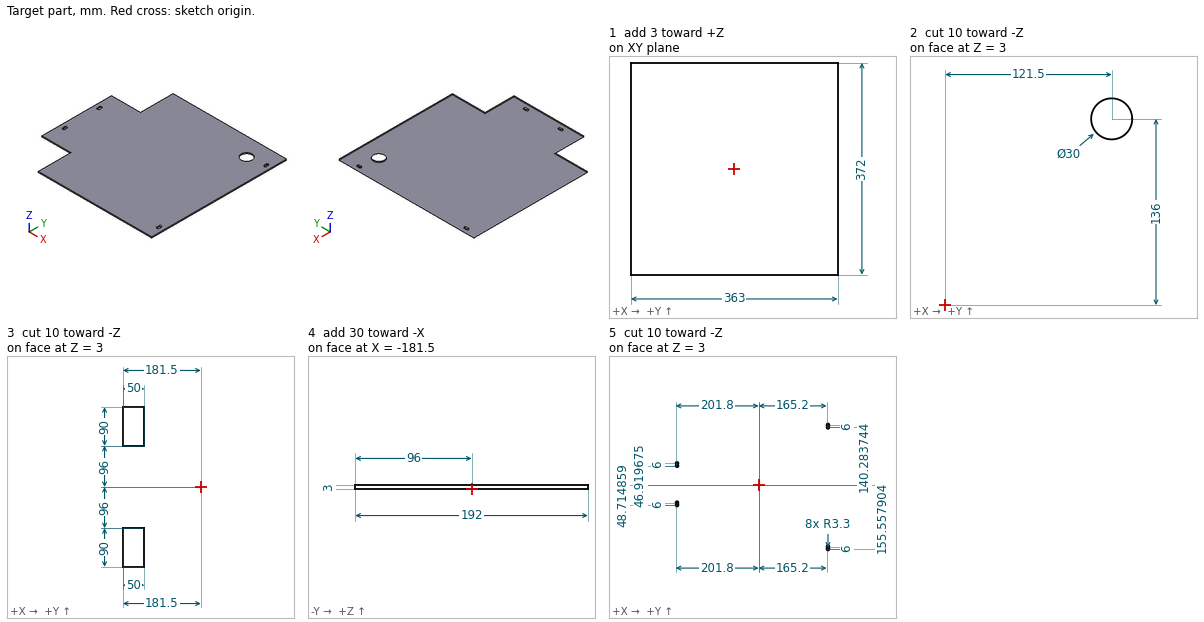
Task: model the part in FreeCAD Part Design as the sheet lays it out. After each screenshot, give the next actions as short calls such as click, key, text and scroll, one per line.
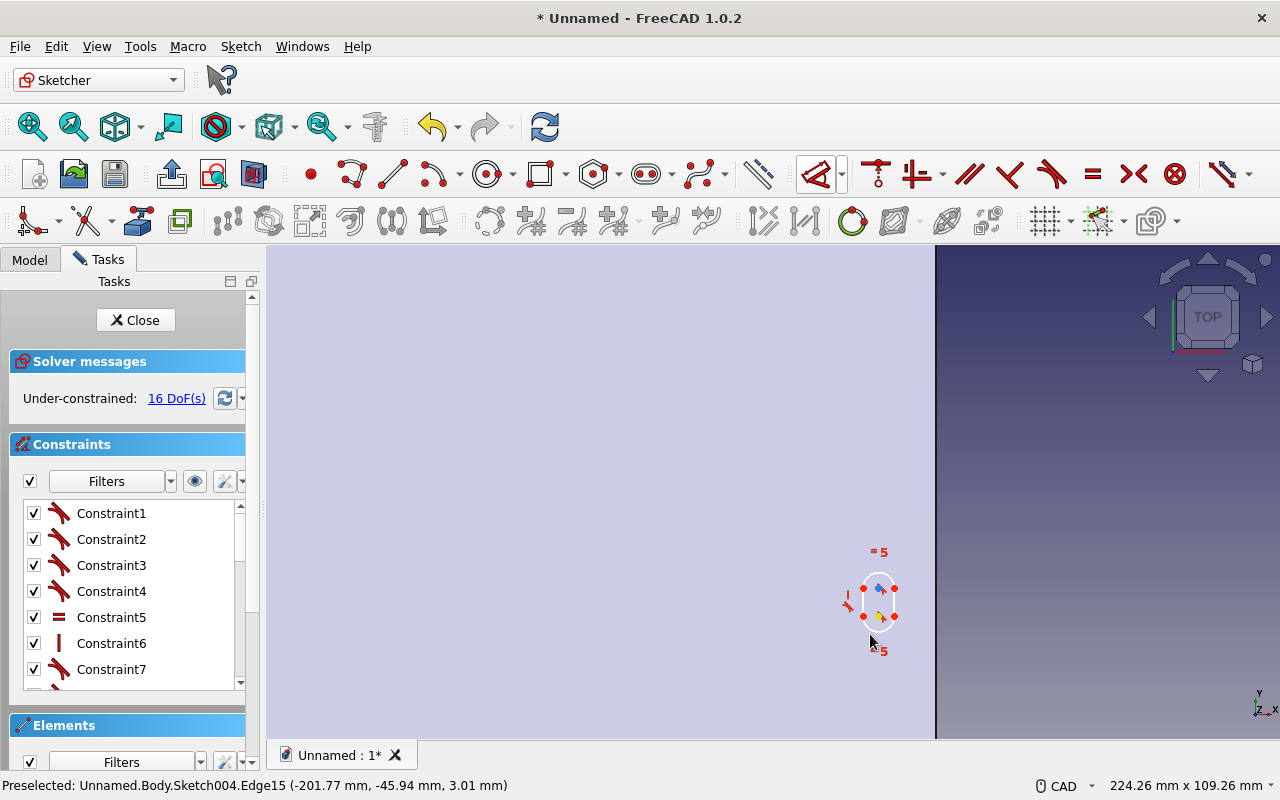
click(870, 629)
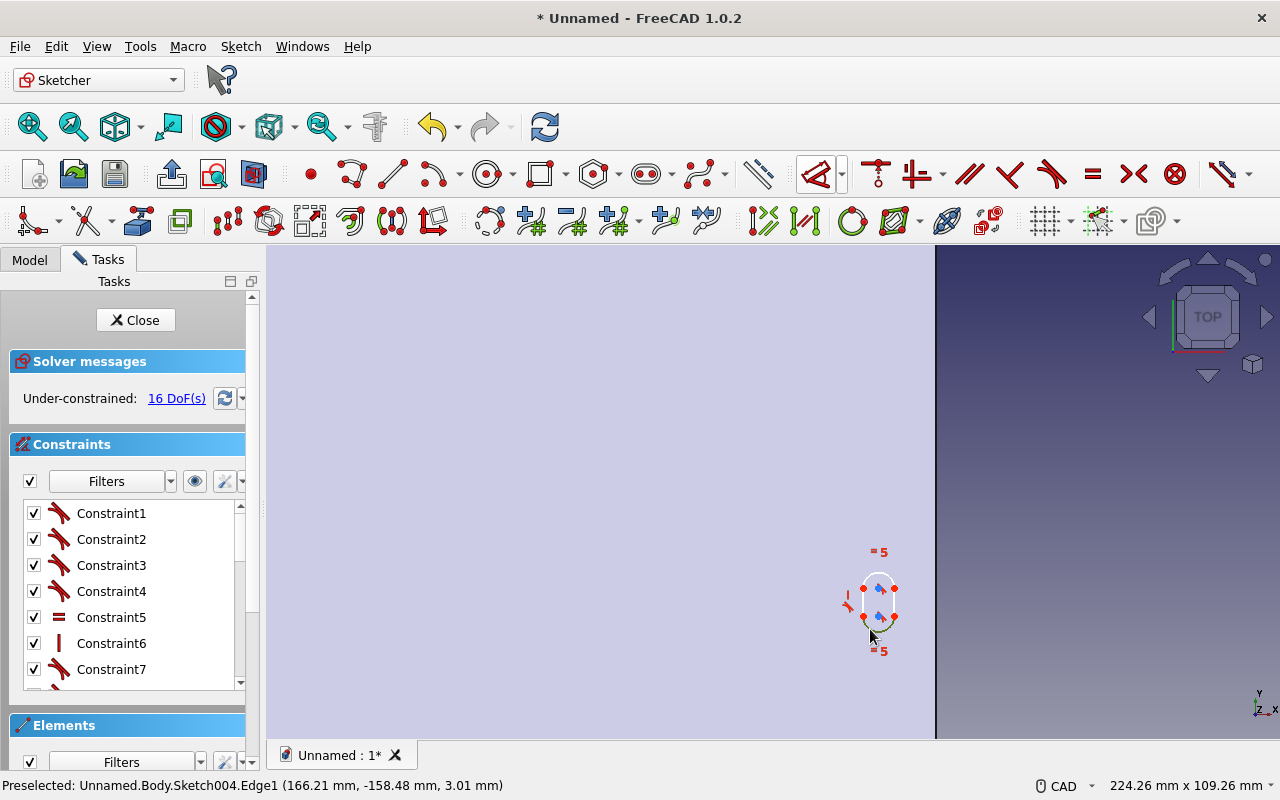
scroll(871, 634, down, 8)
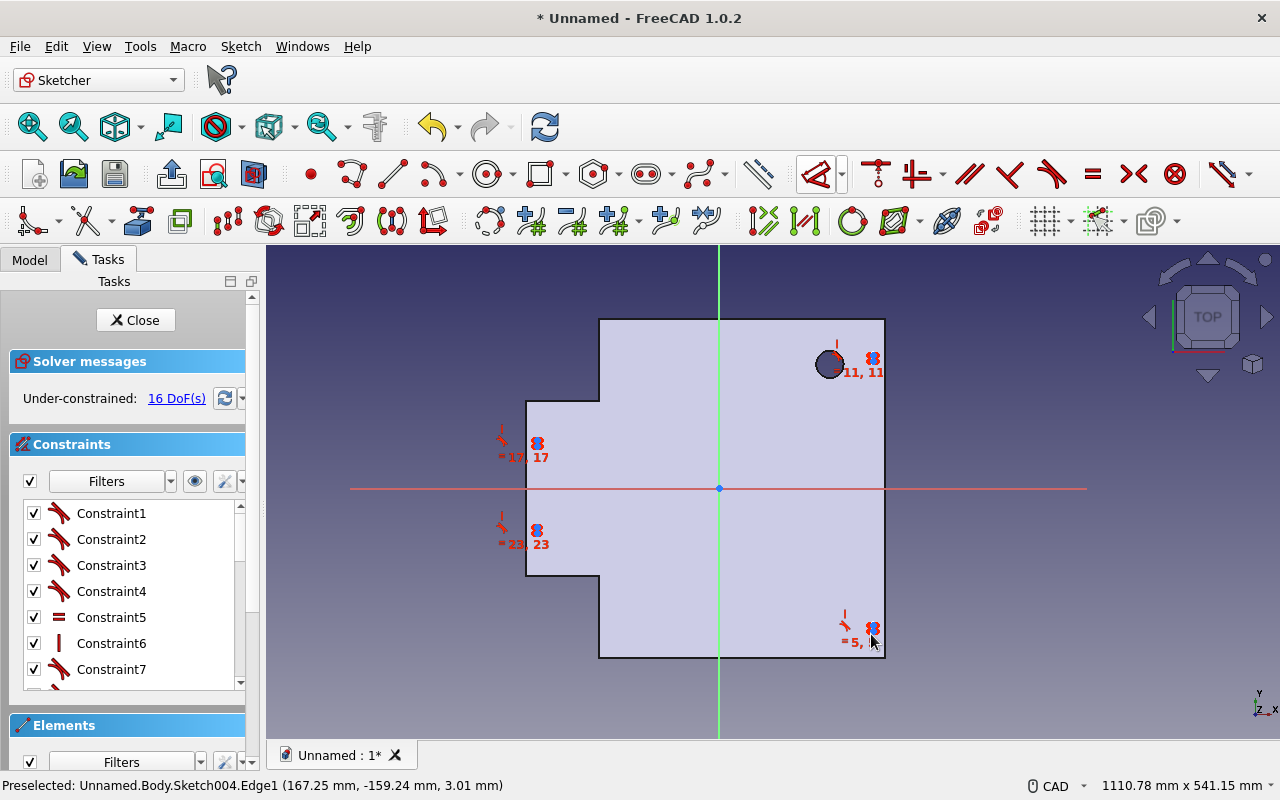
scroll(871, 364, up, 8)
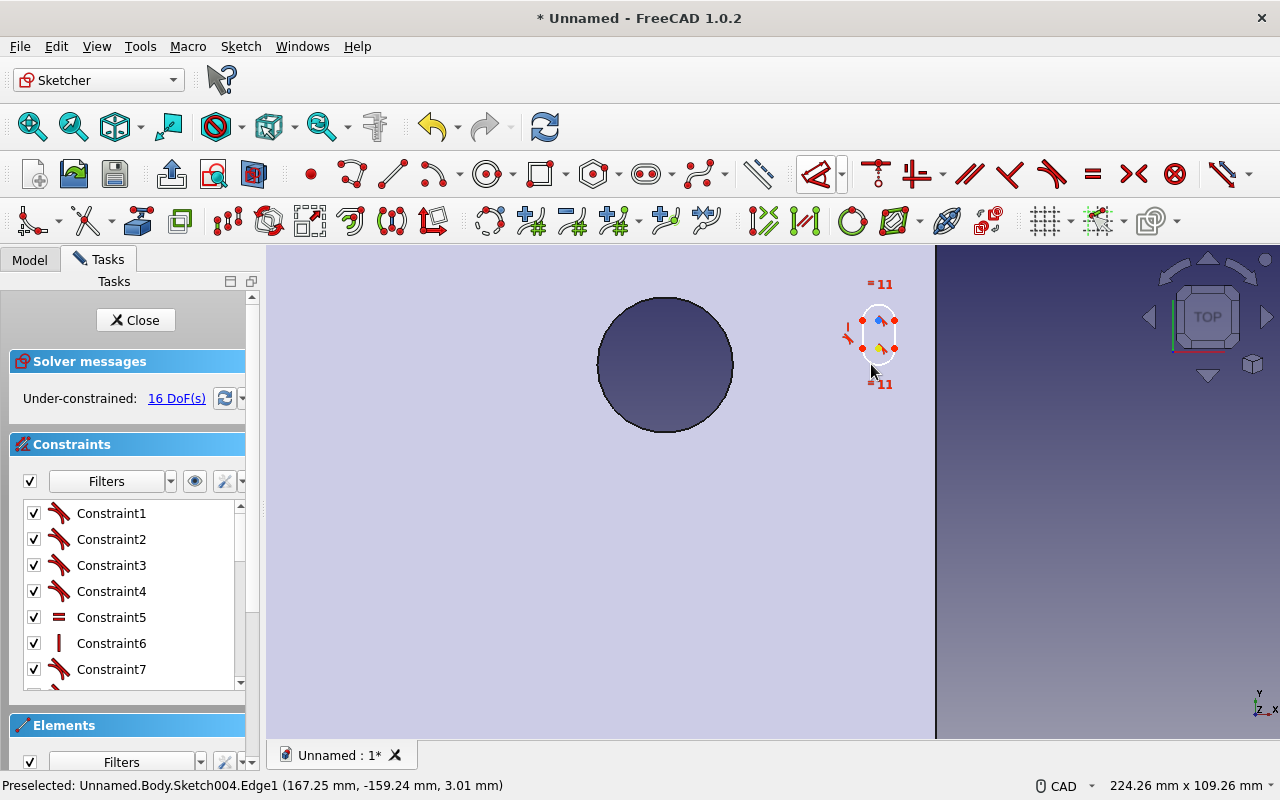
click(869, 362)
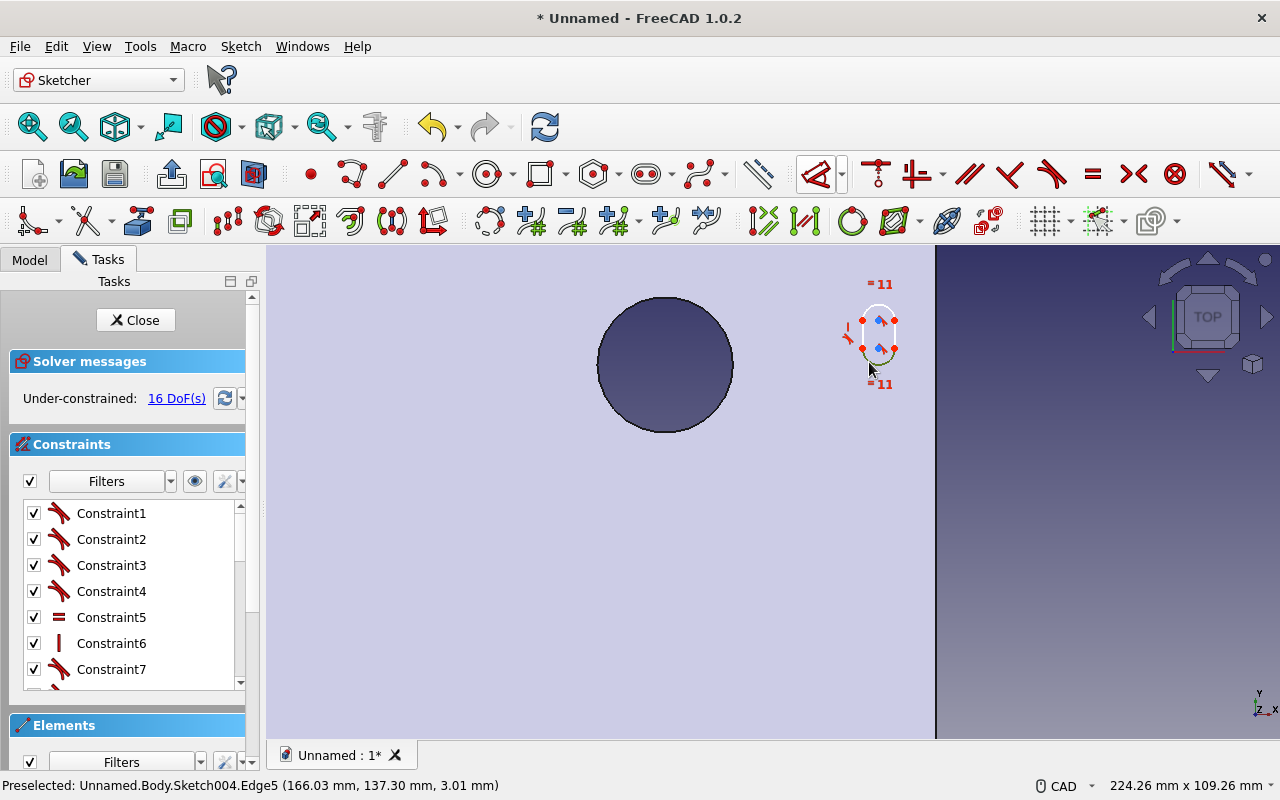
scroll(871, 363, down, 8)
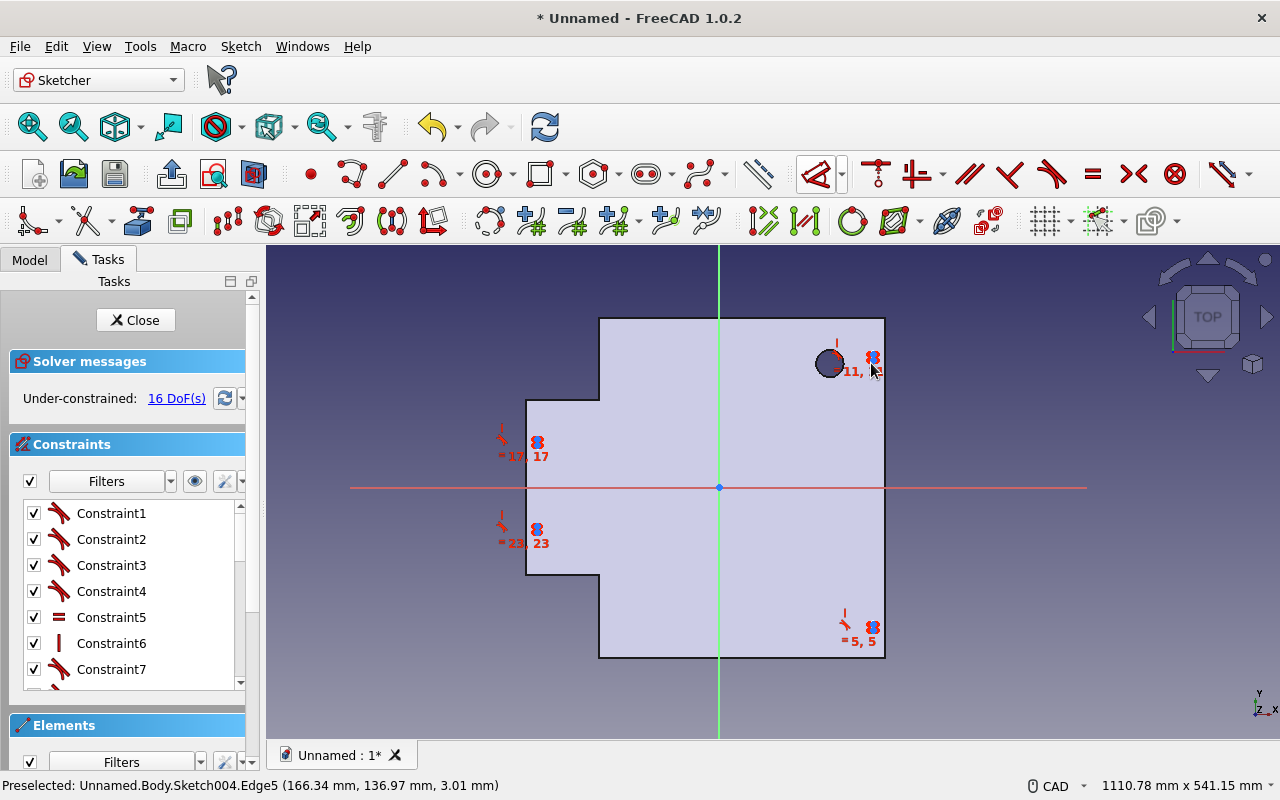
scroll(536, 448, up, 9)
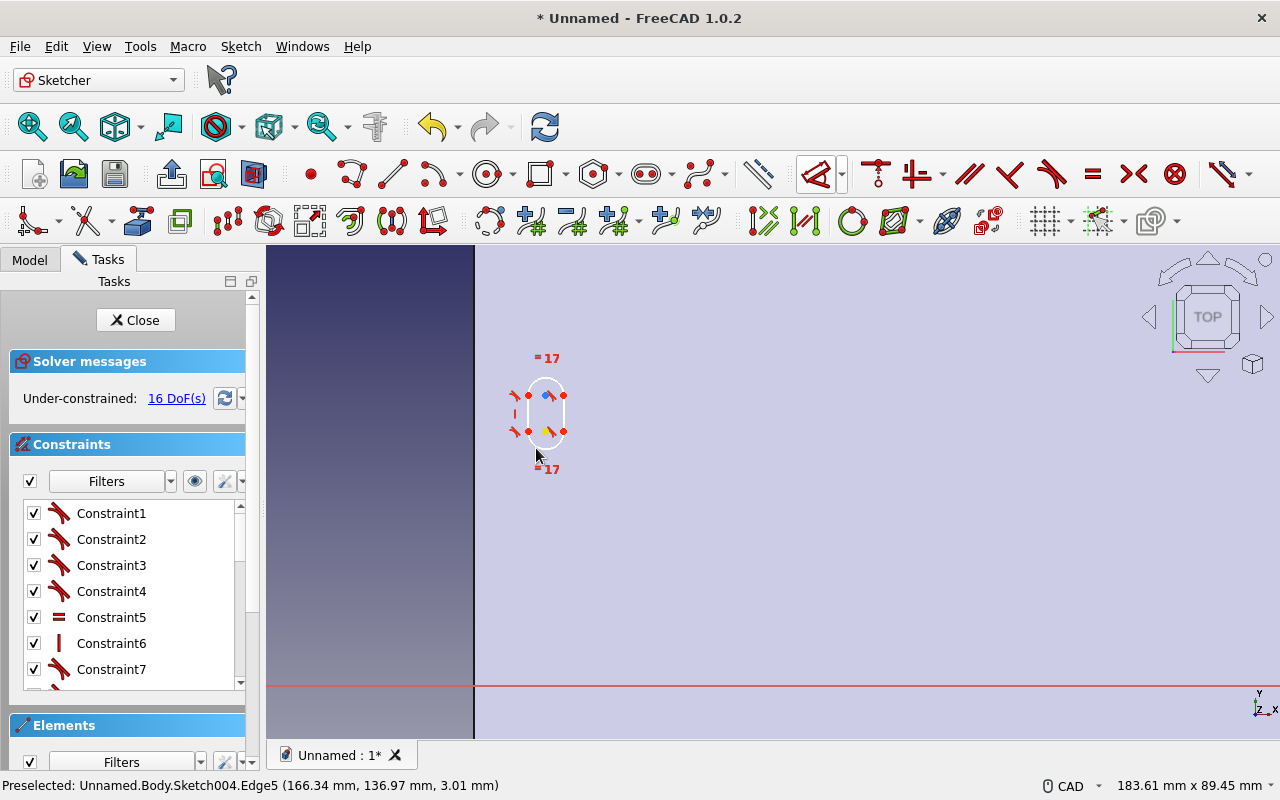
click(535, 446)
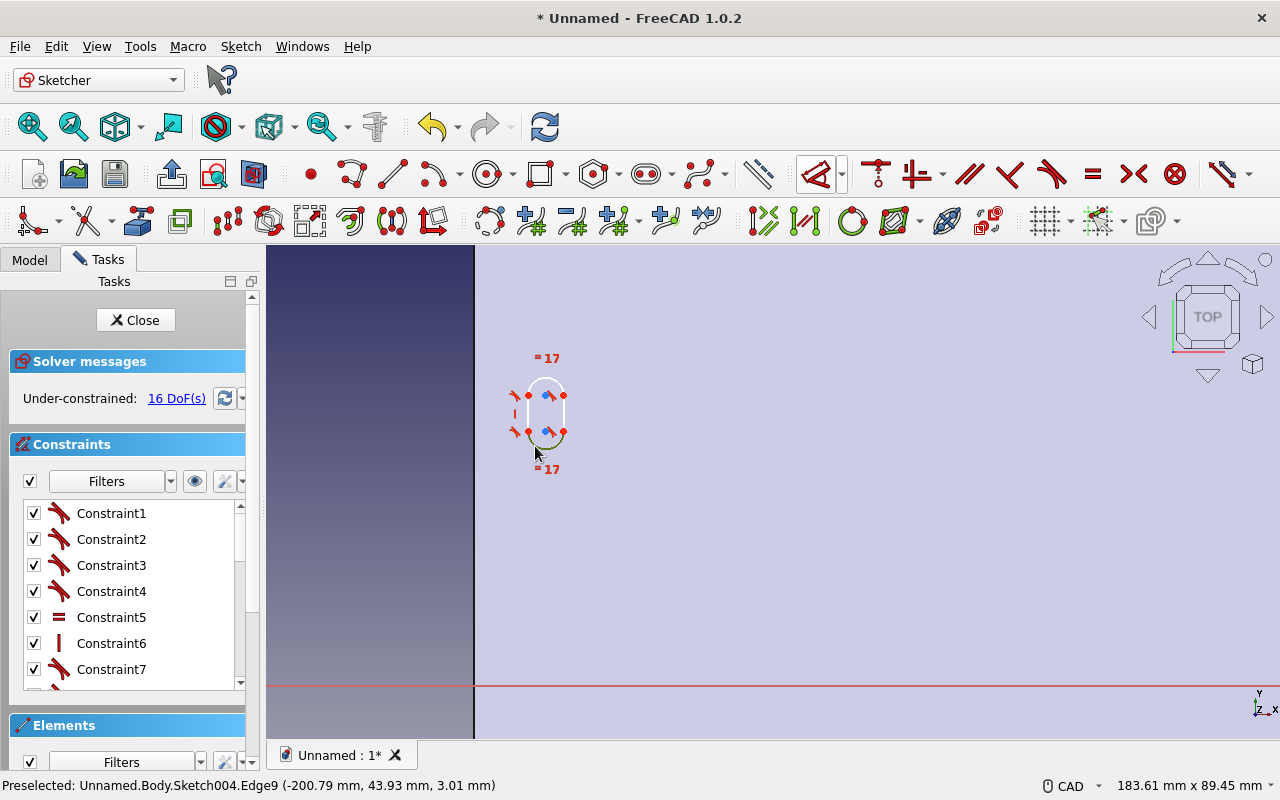
scroll(535, 448, down, 9)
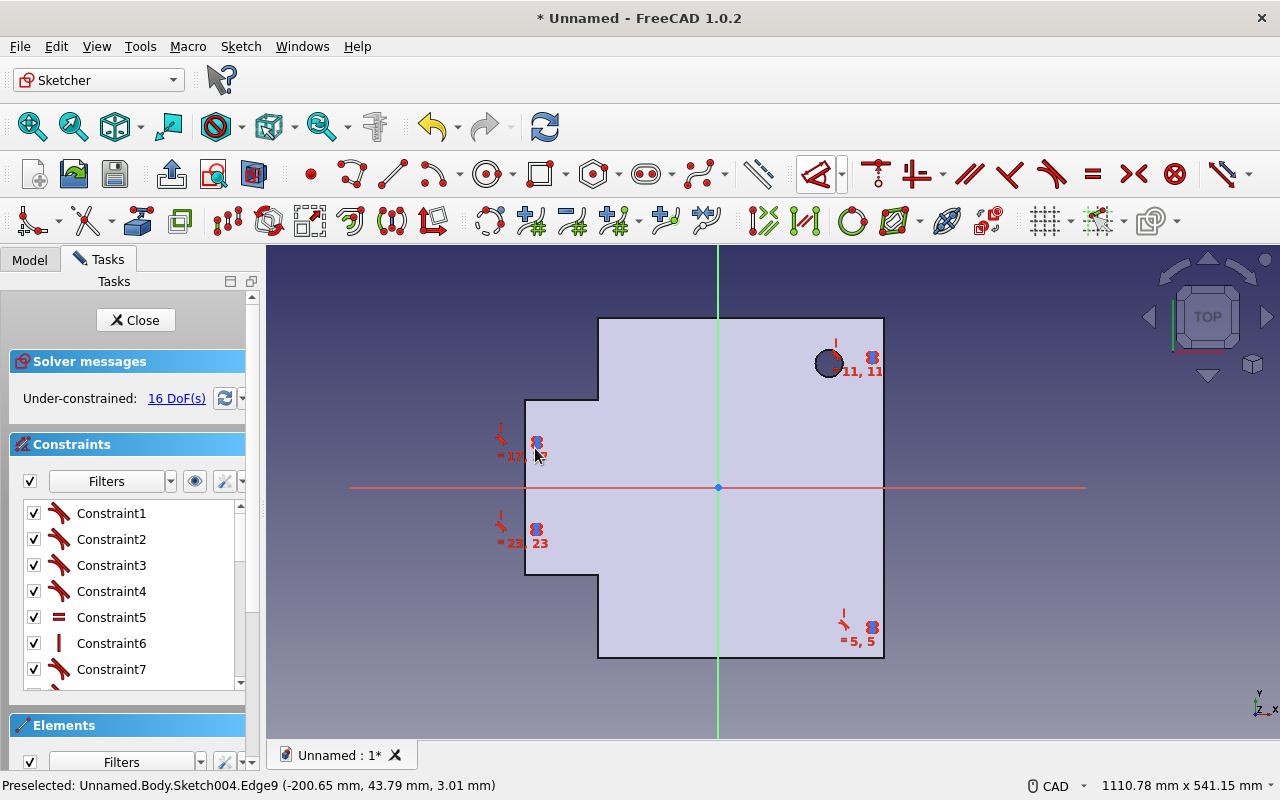
scroll(535, 535, up, 9)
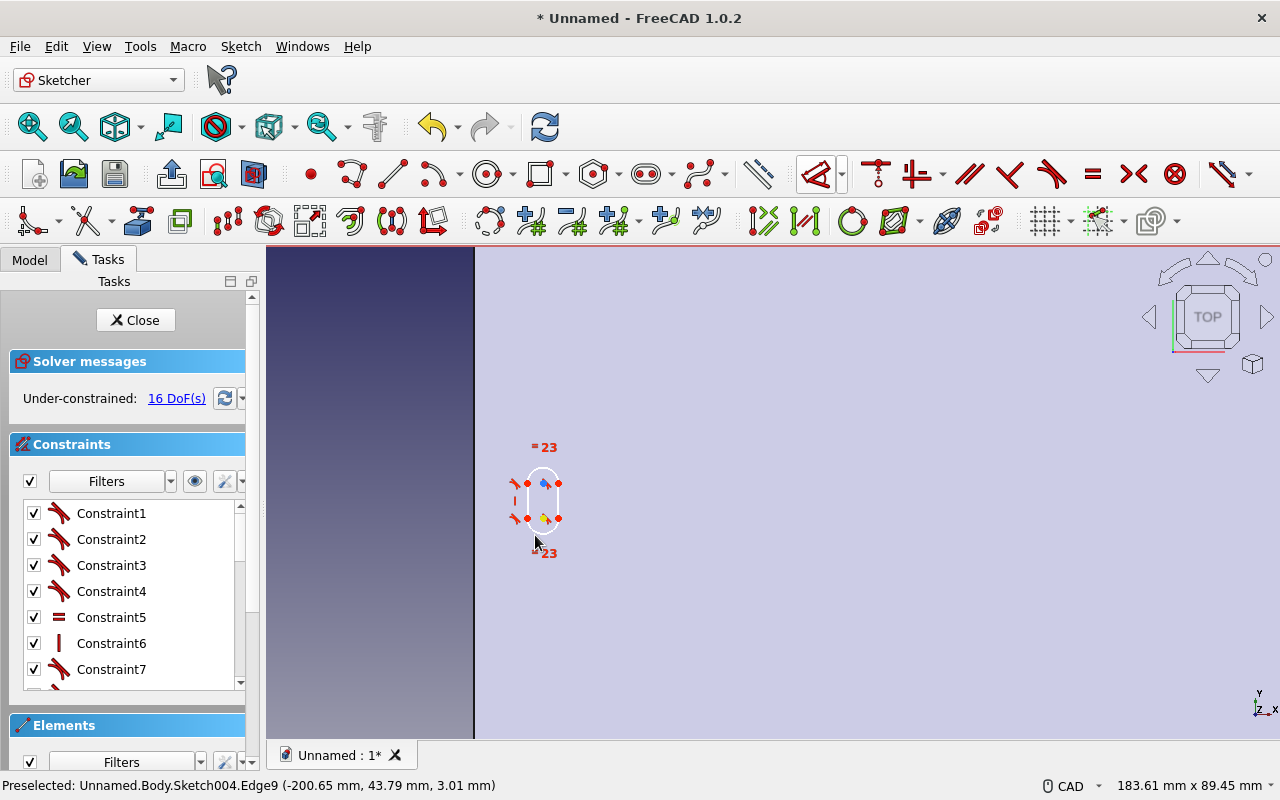
click(534, 531)